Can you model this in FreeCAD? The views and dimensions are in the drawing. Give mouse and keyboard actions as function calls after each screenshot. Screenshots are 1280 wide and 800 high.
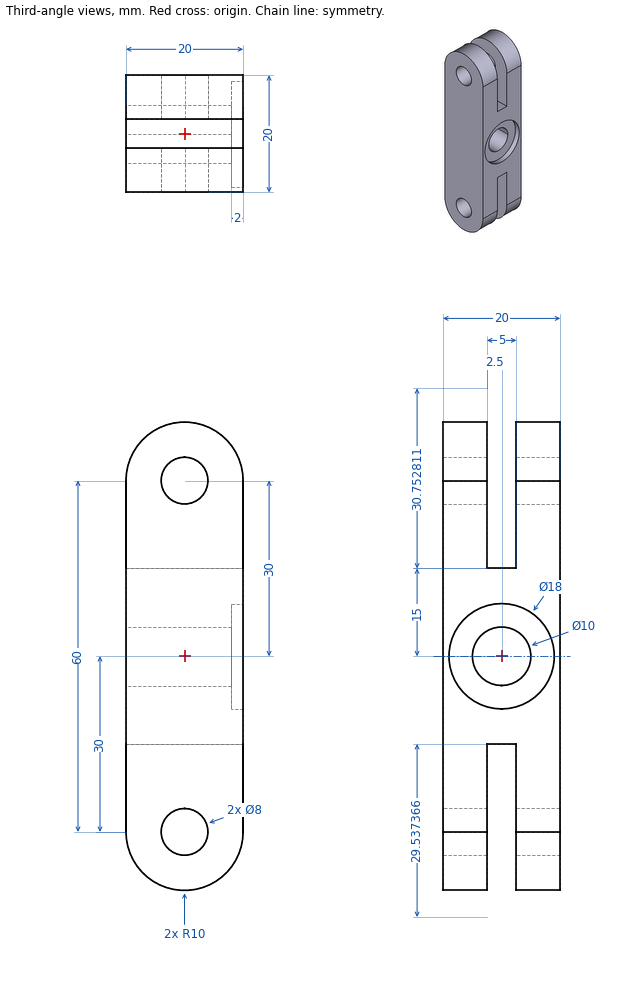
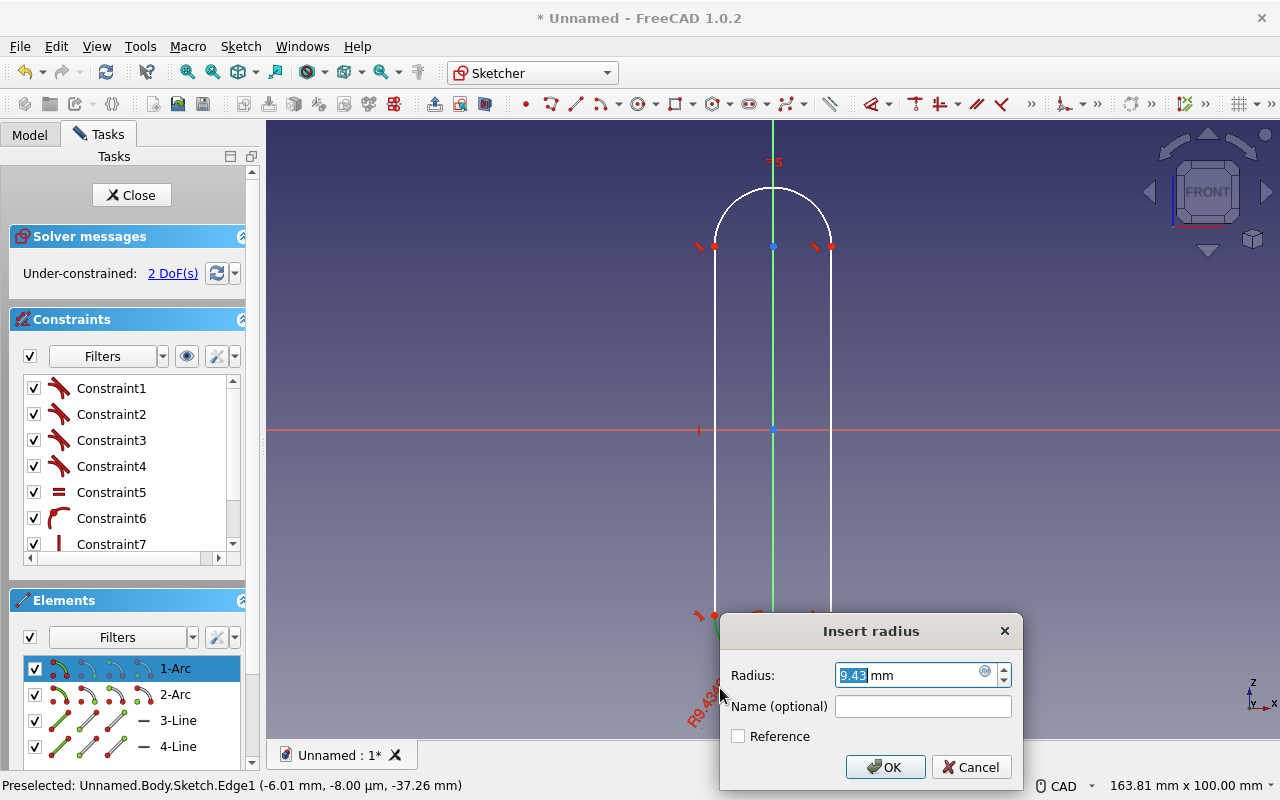
text(10)
key(Return)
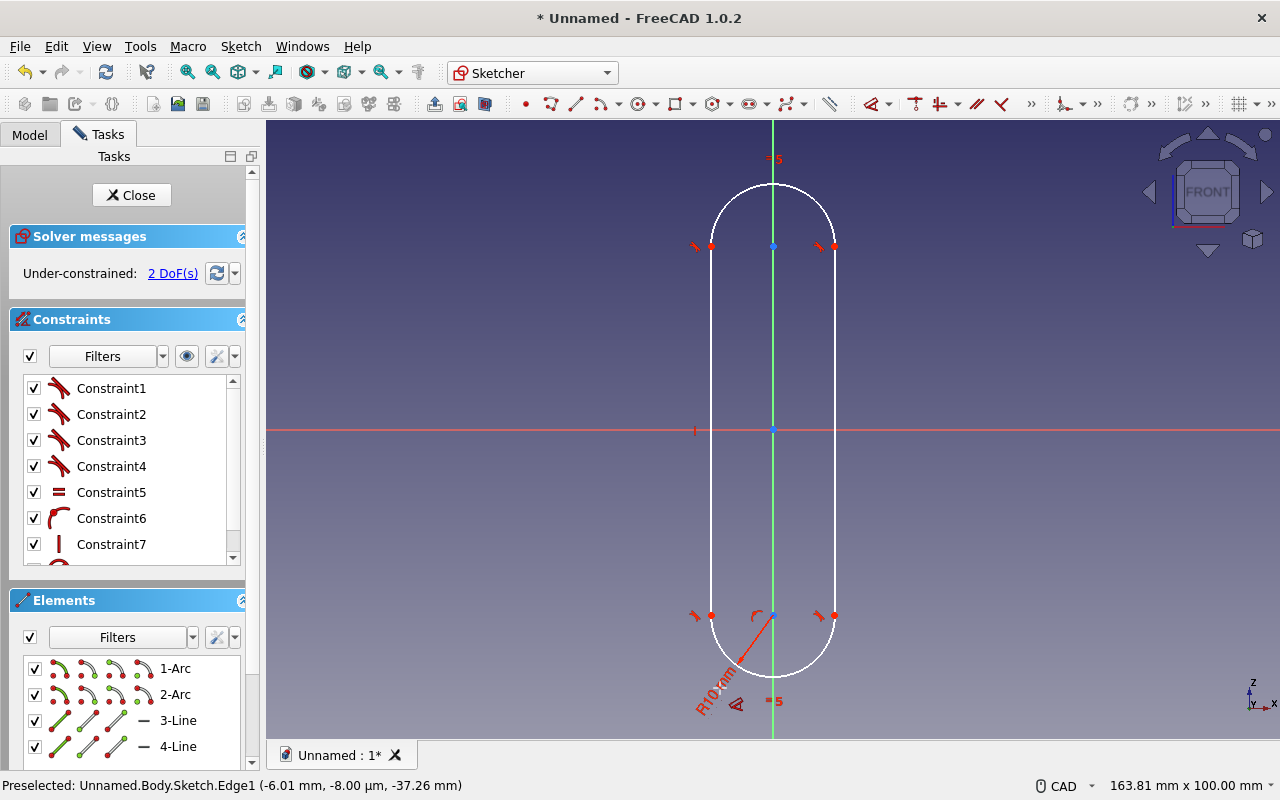
click(711, 504)
click(677, 346)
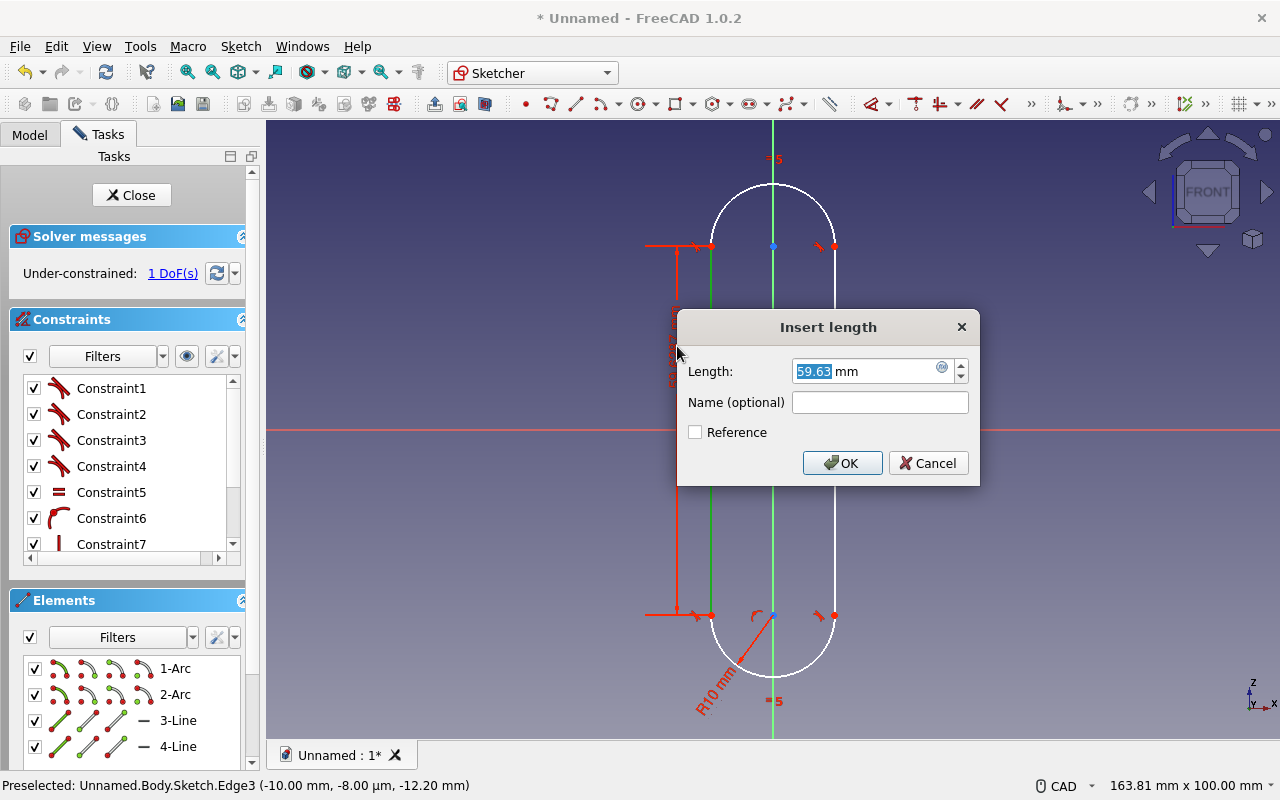
text(60)
key(Return)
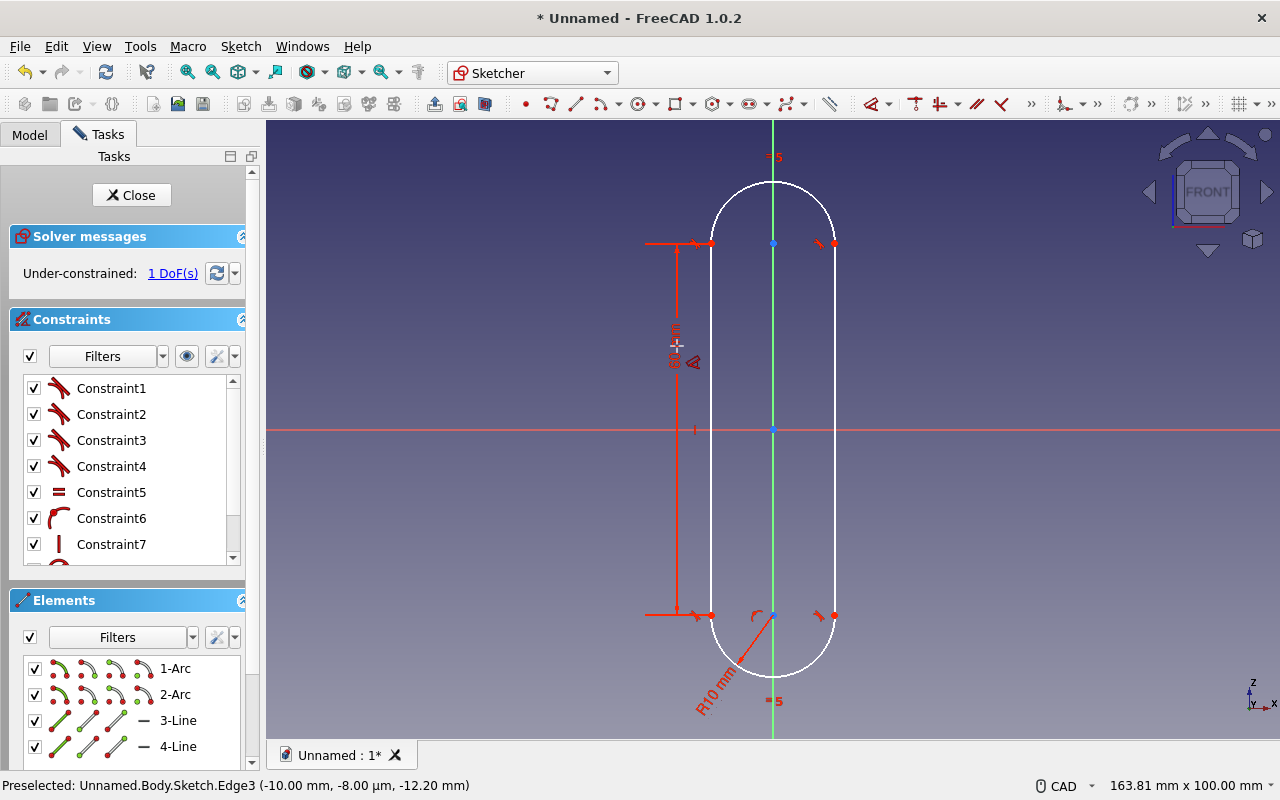
click(711, 615)
click(677, 522)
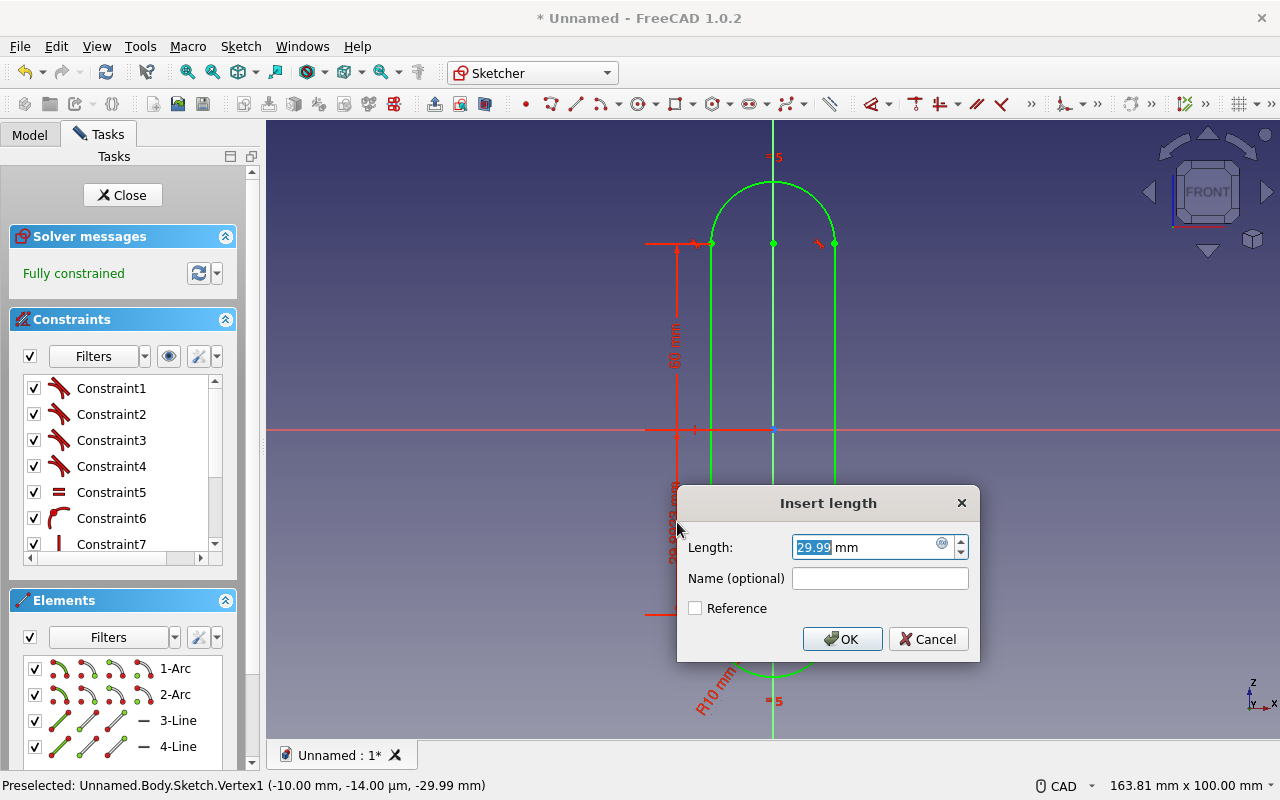
text(30)
key(Return)
key(Escape)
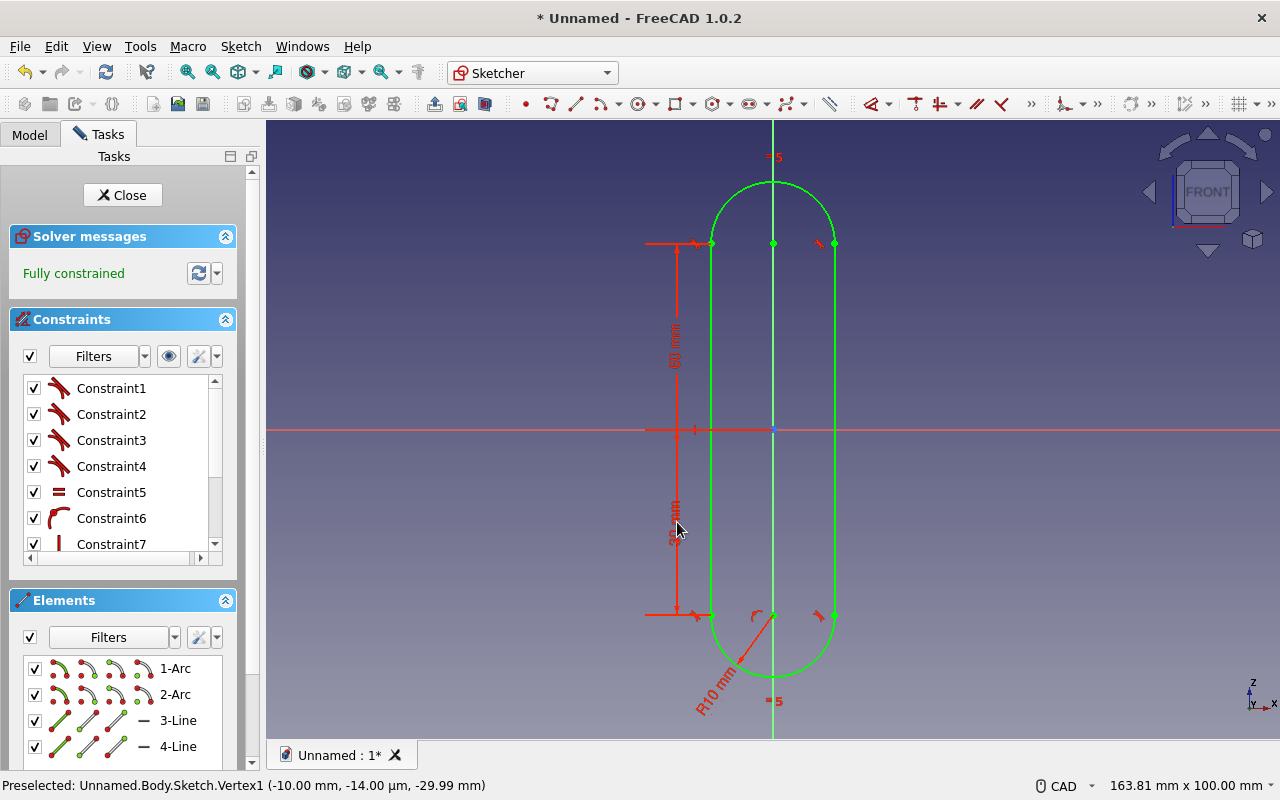
click(123, 195)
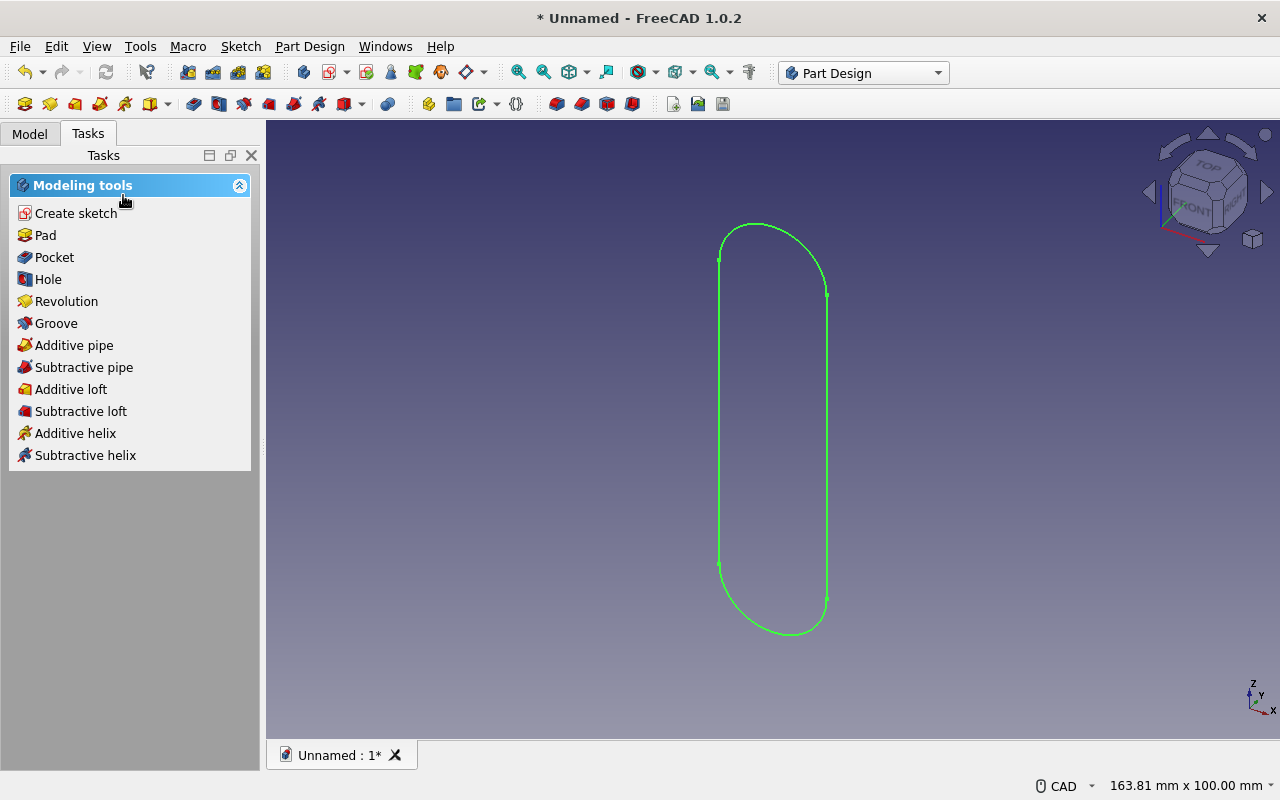
click(25, 104)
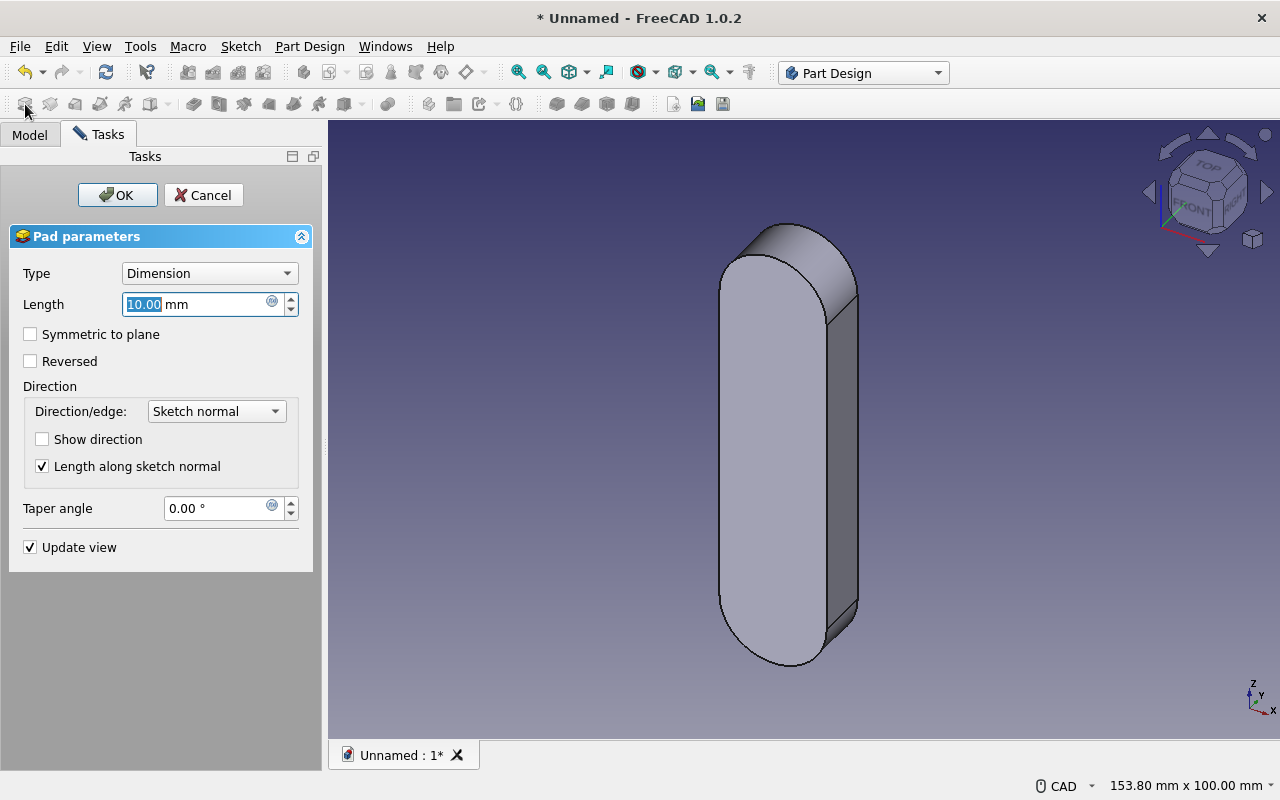
text(20)
key(Tab)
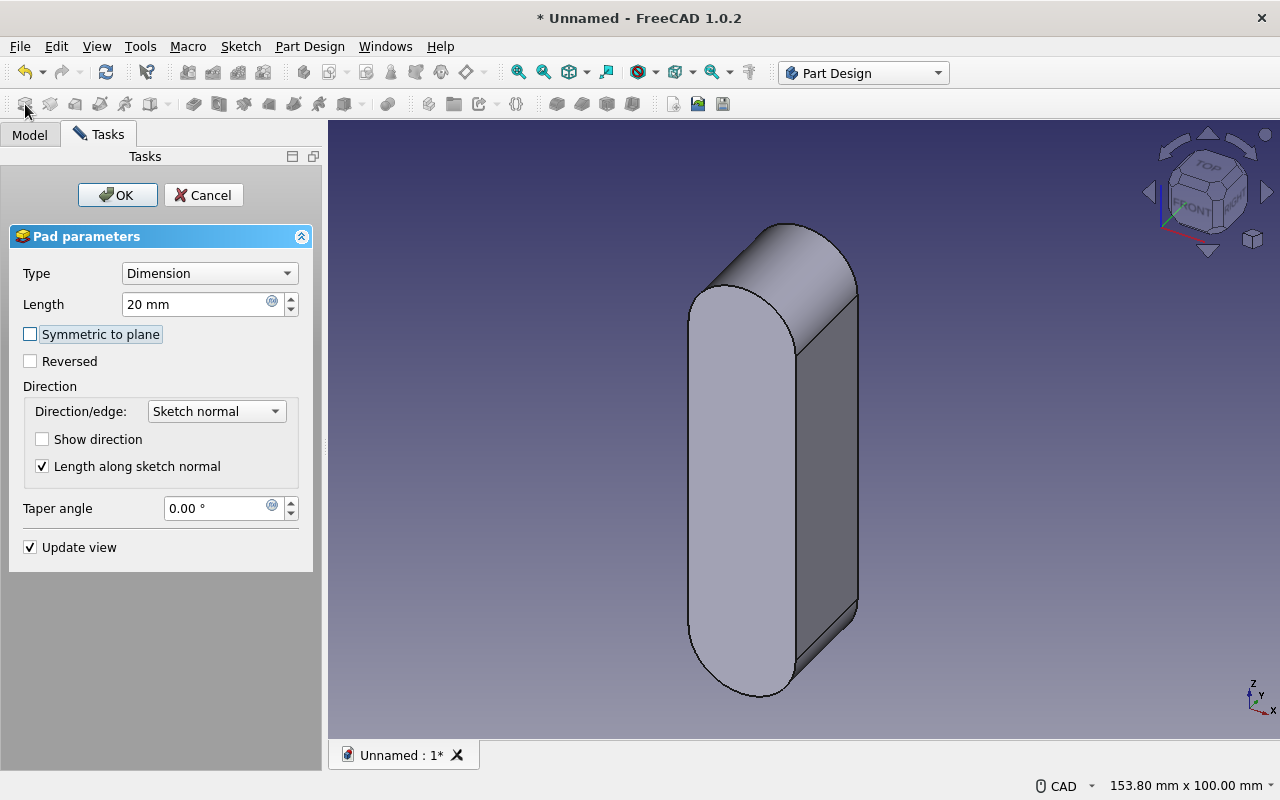
click(31, 334)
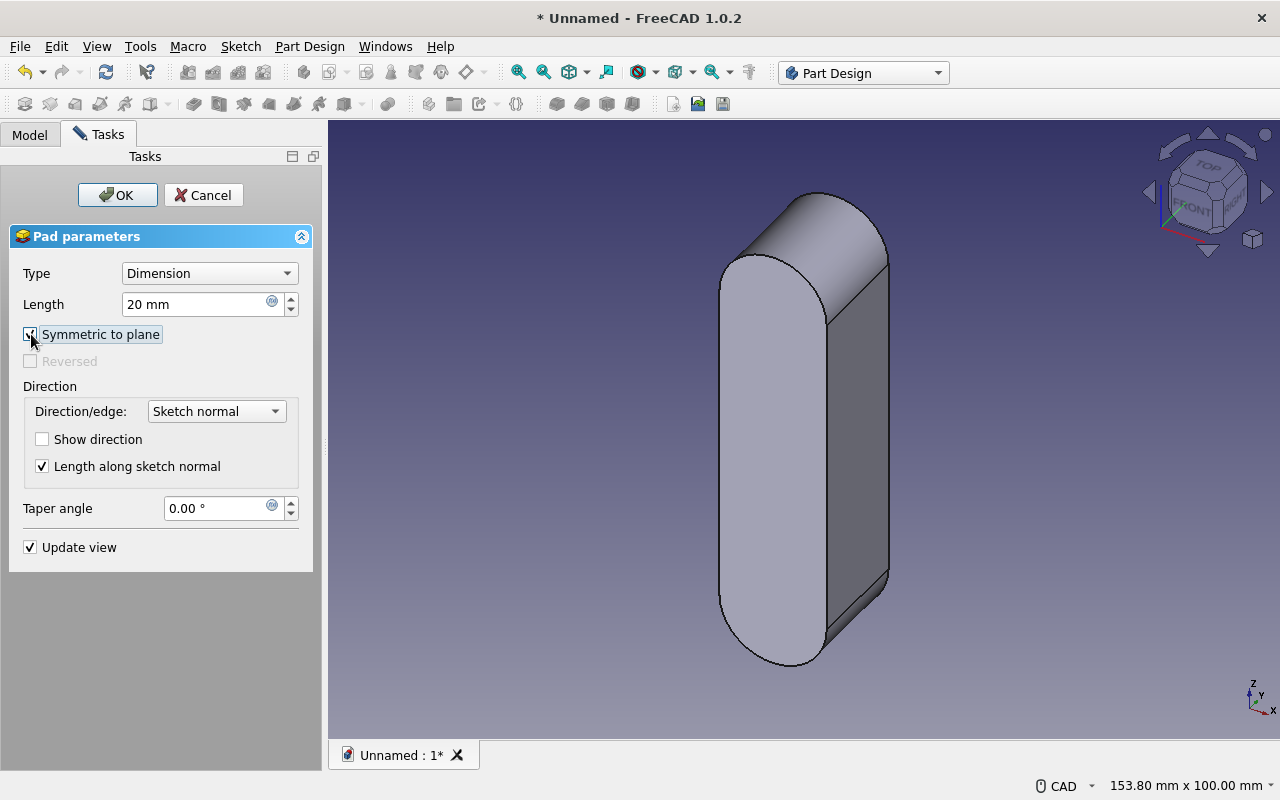
click(118, 195)